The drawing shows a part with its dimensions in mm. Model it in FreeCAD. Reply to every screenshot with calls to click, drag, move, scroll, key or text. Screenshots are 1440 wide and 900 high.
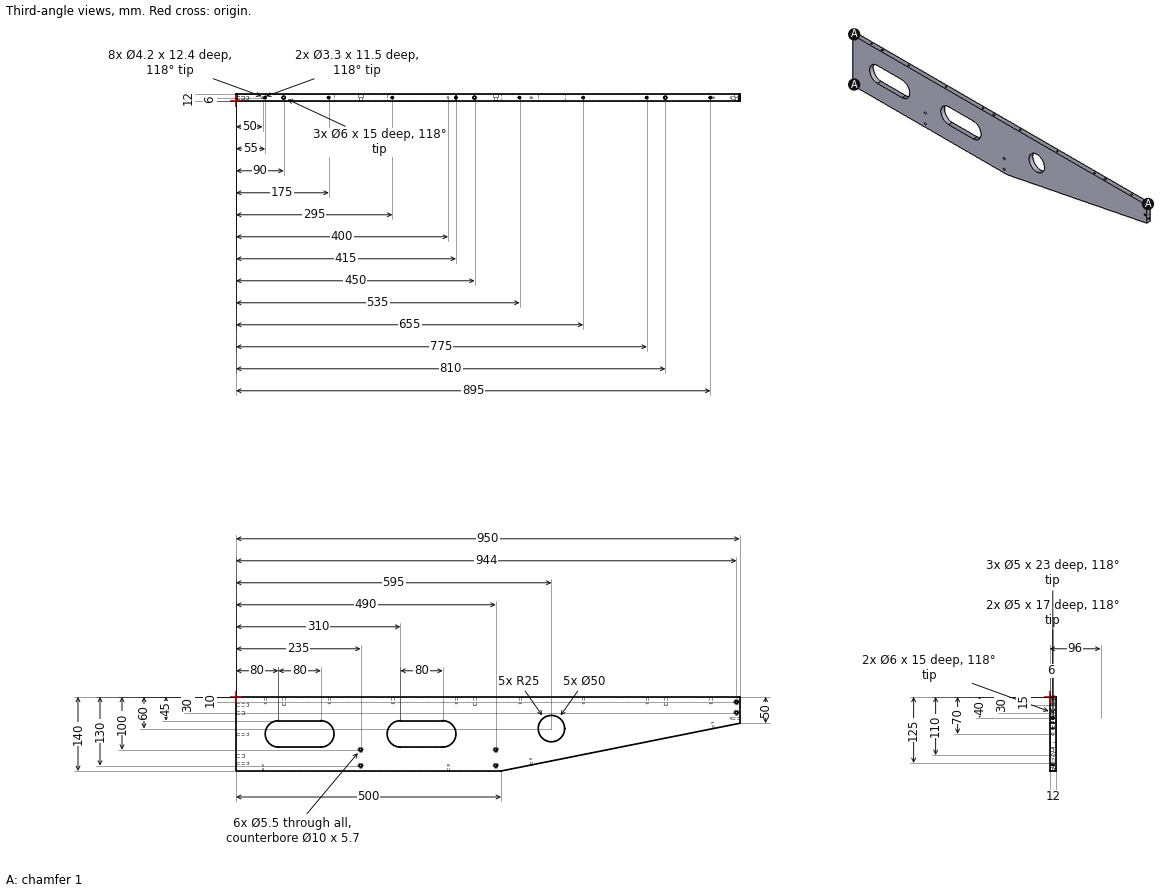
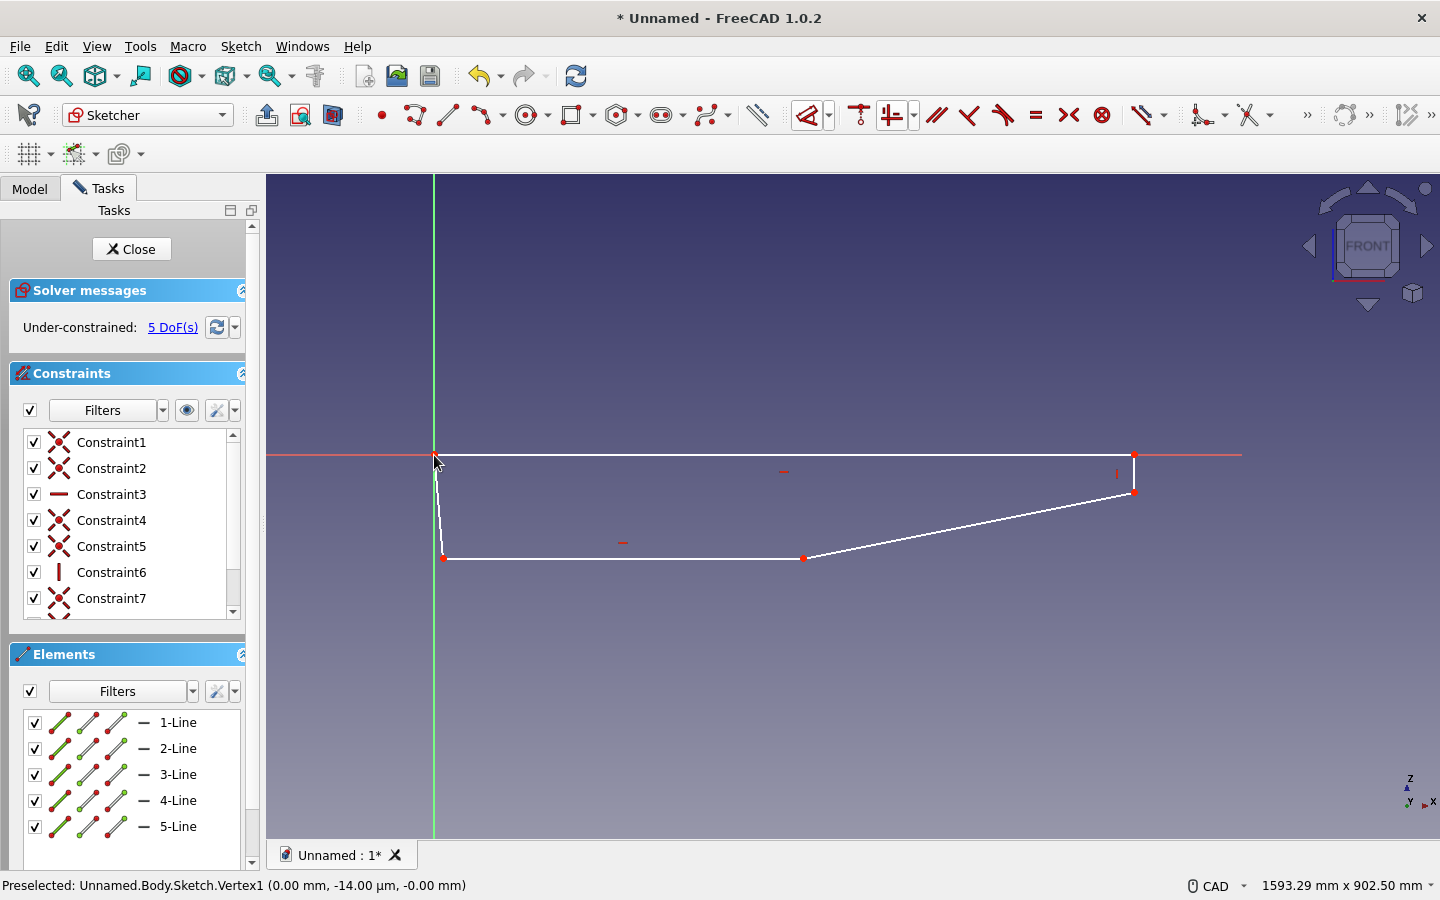
click(437, 486)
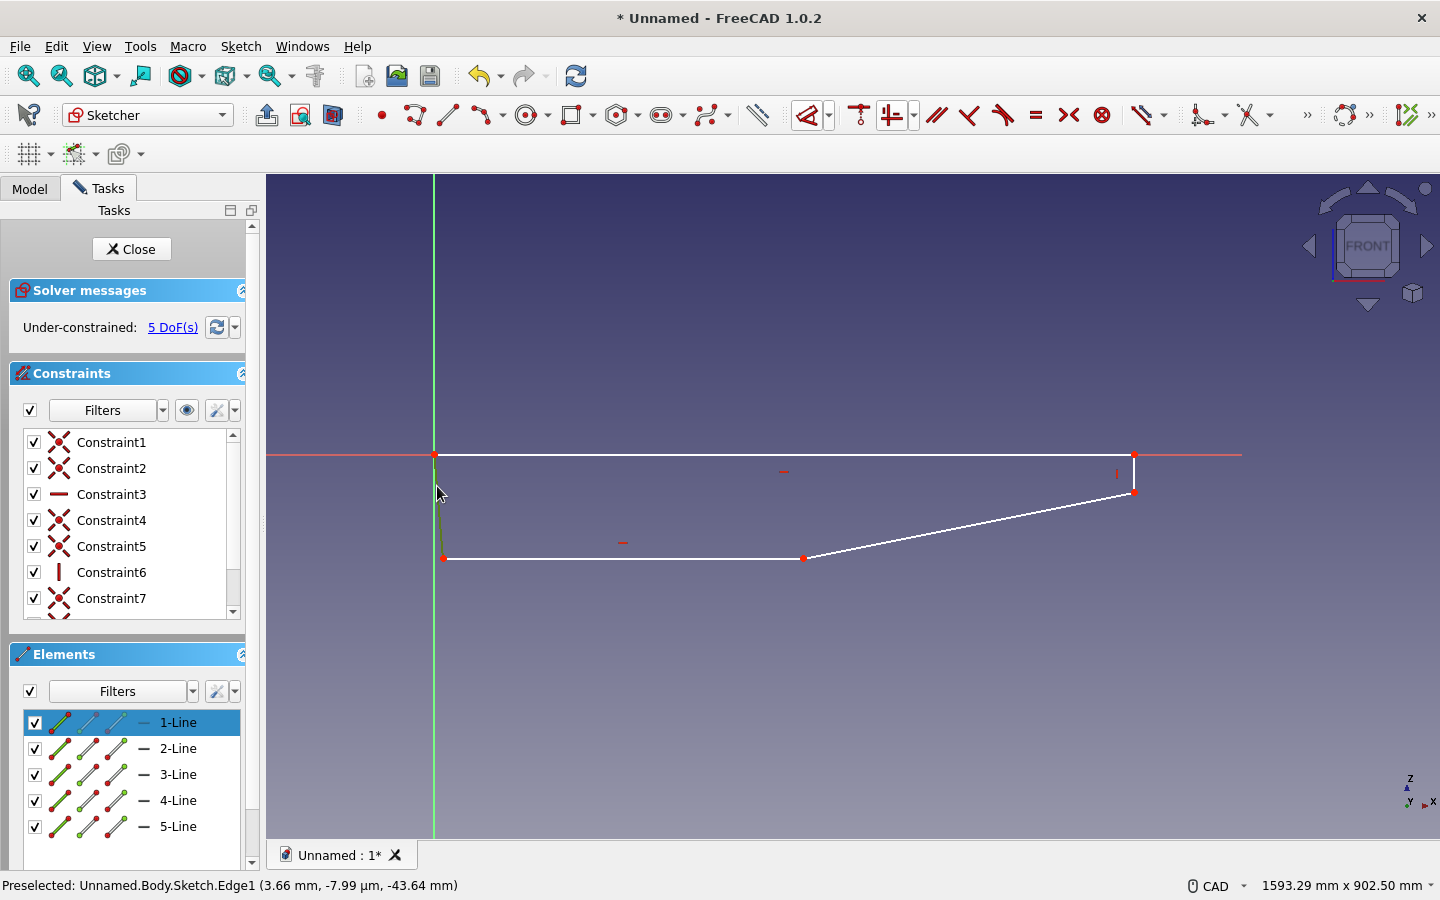
key(v)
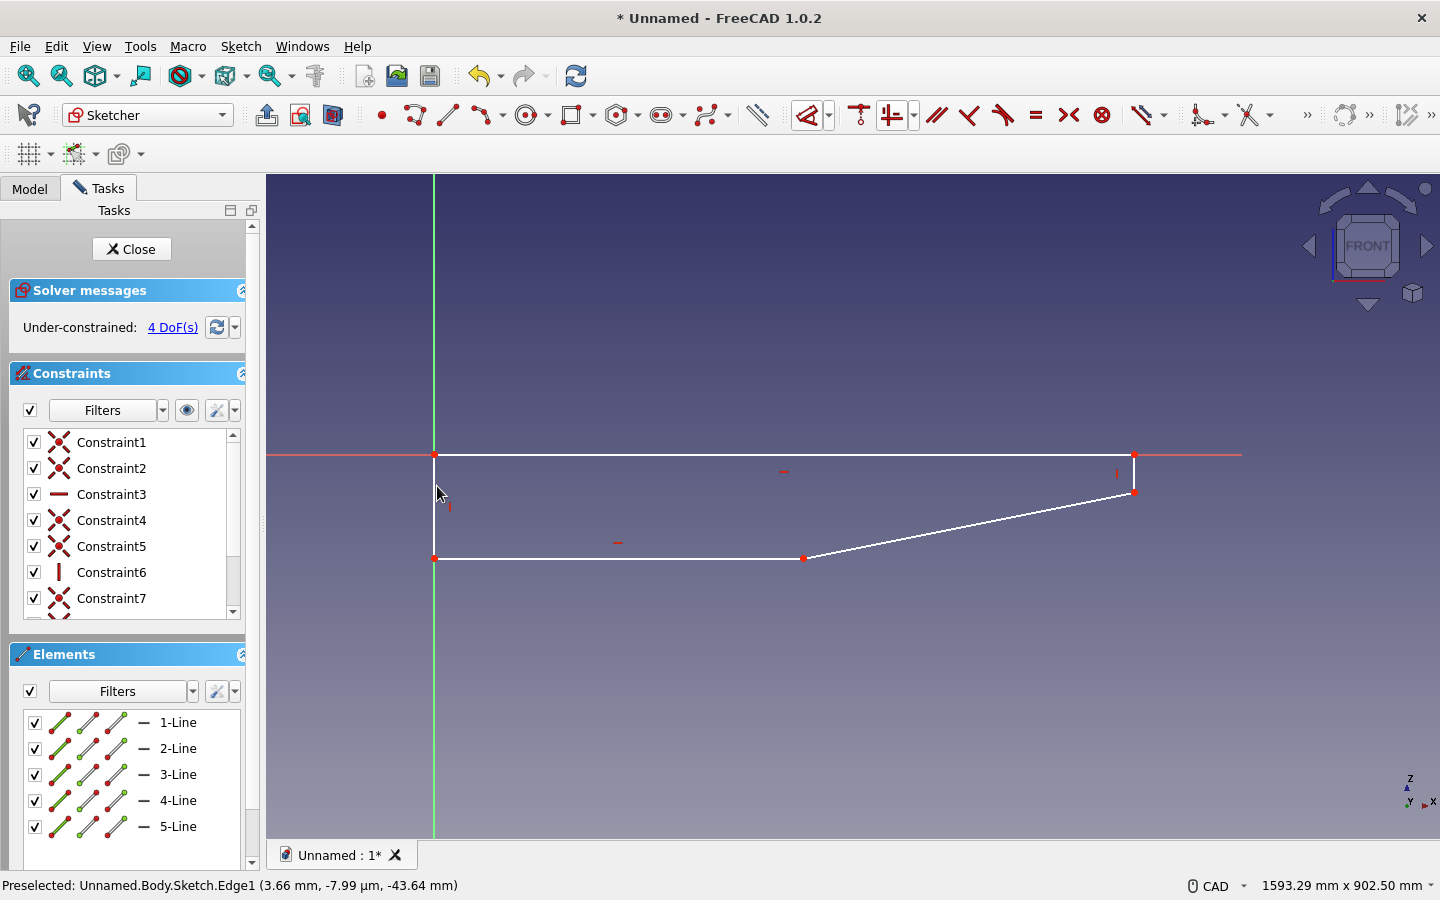
click(806, 116)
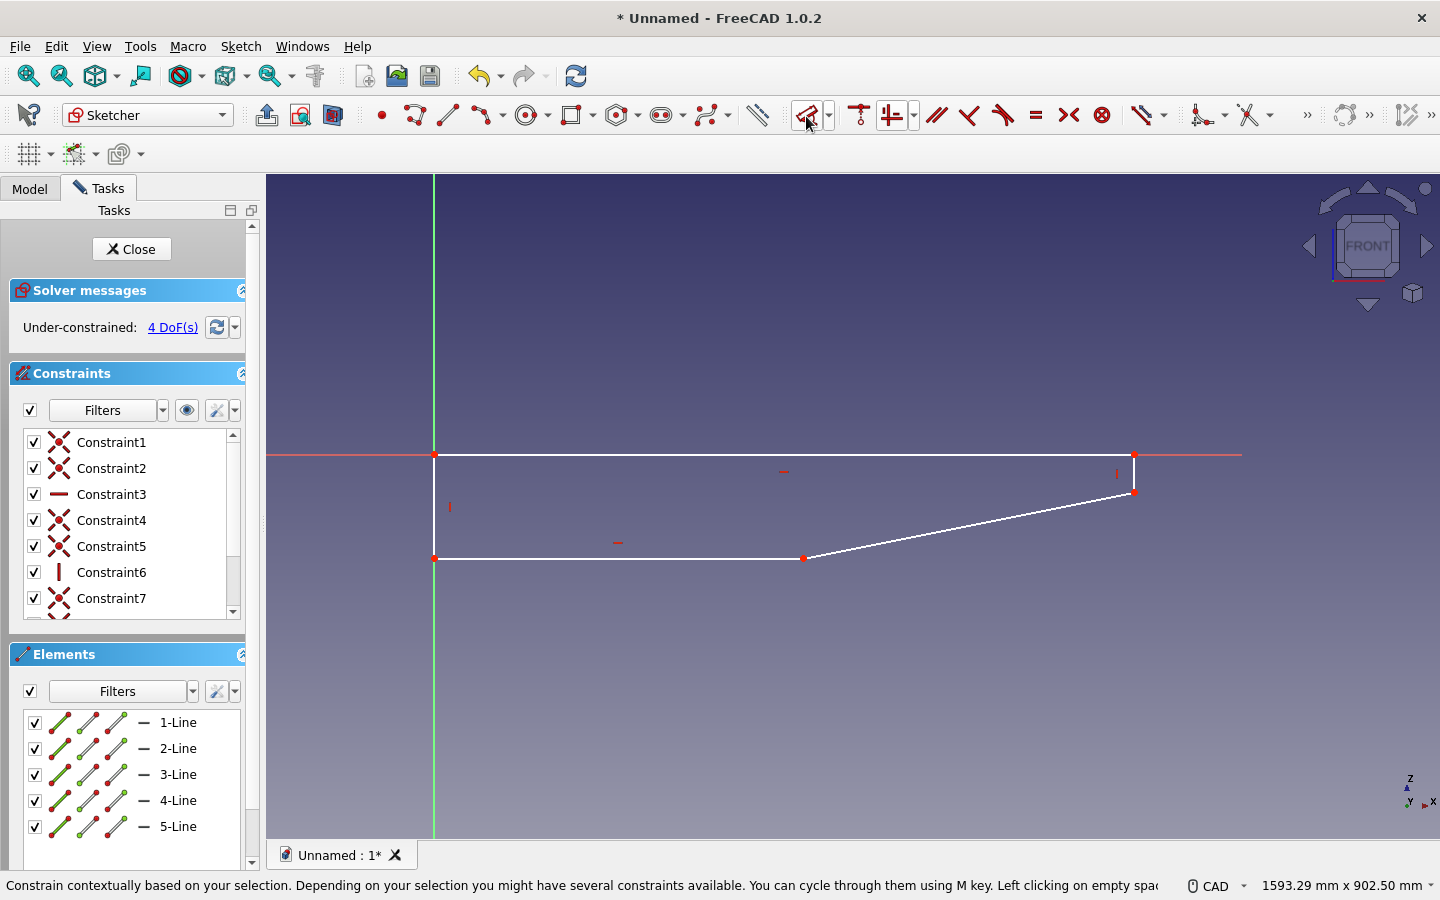
click(1134, 482)
click(1168, 474)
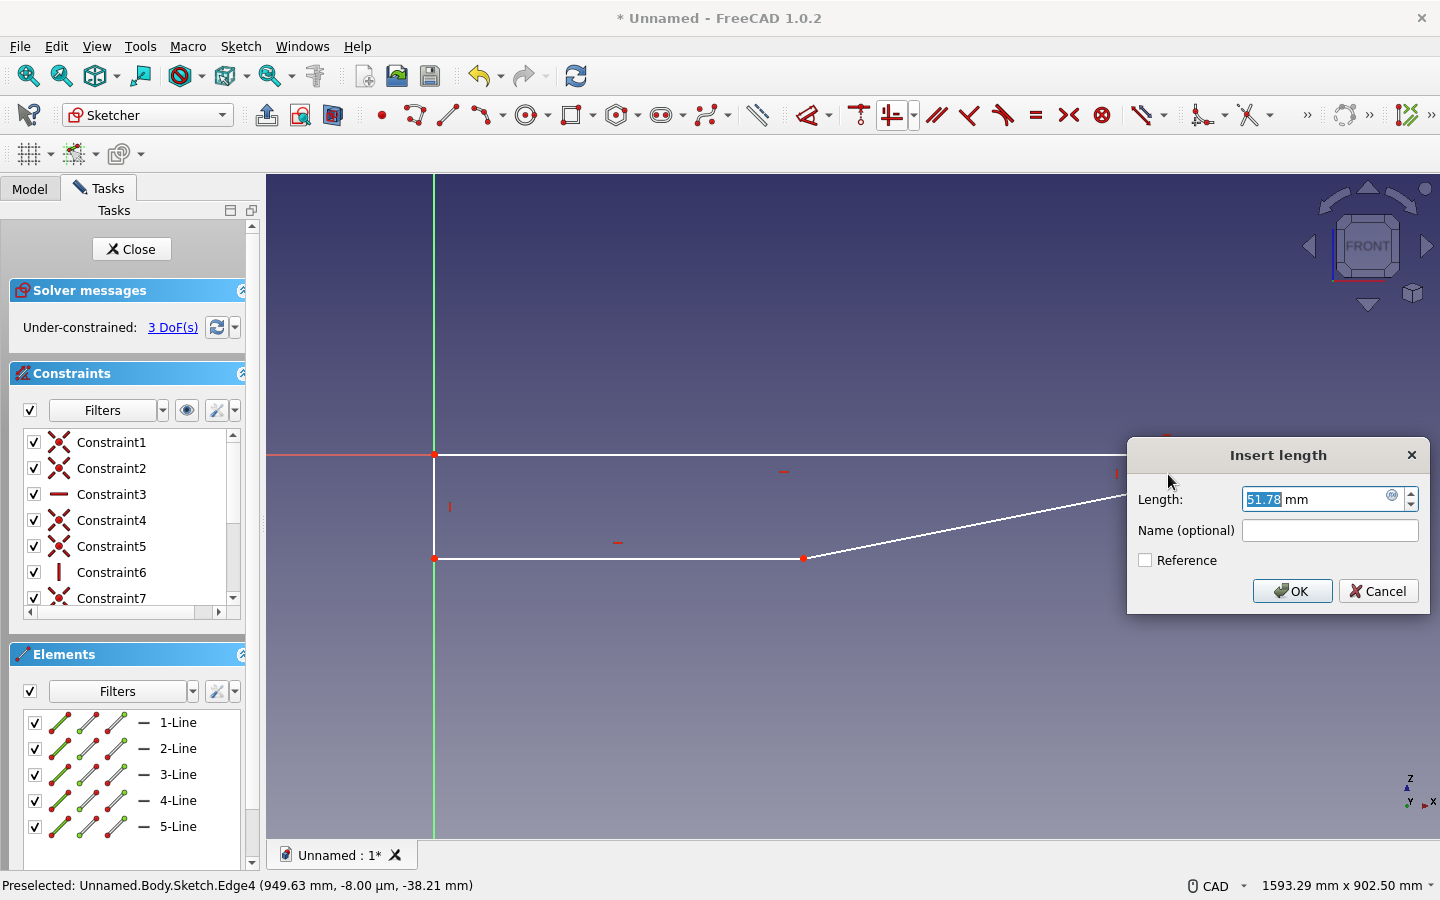
text(50)
key(Return)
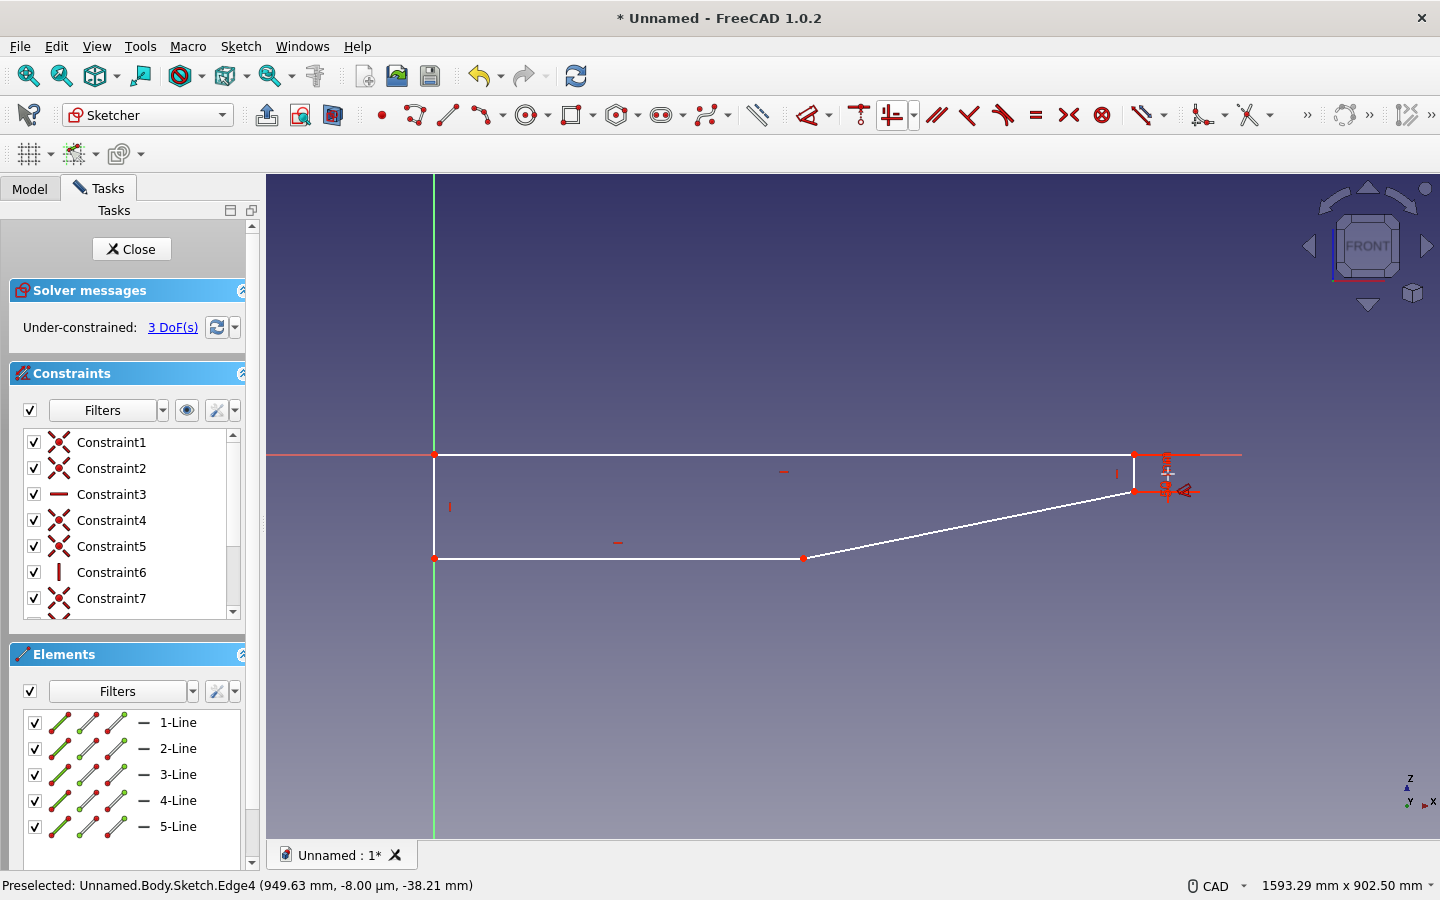
click(434, 486)
click(400, 507)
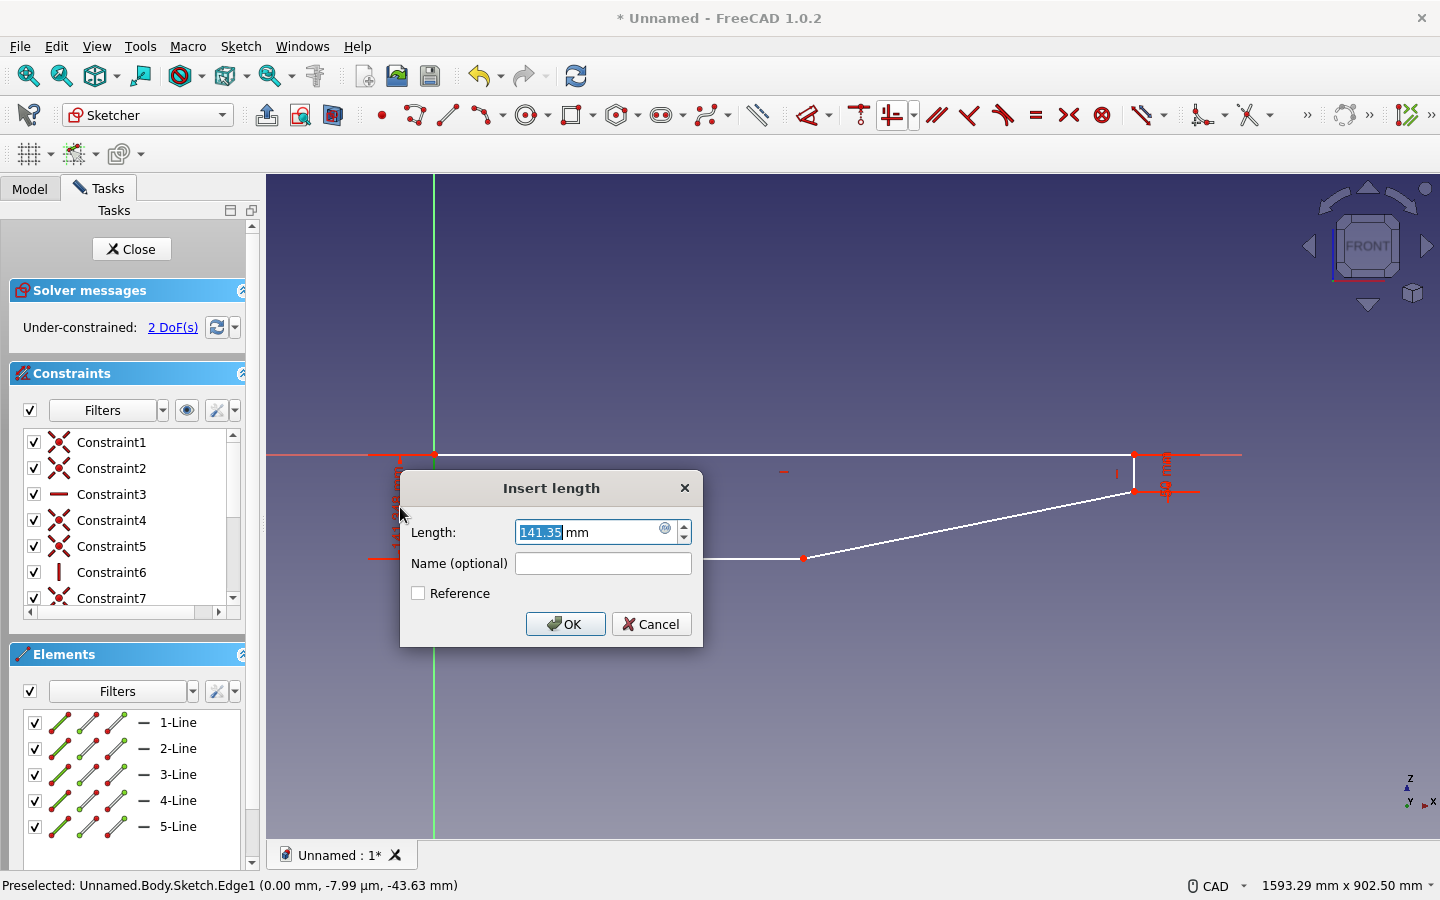
text(140)
key(Return)